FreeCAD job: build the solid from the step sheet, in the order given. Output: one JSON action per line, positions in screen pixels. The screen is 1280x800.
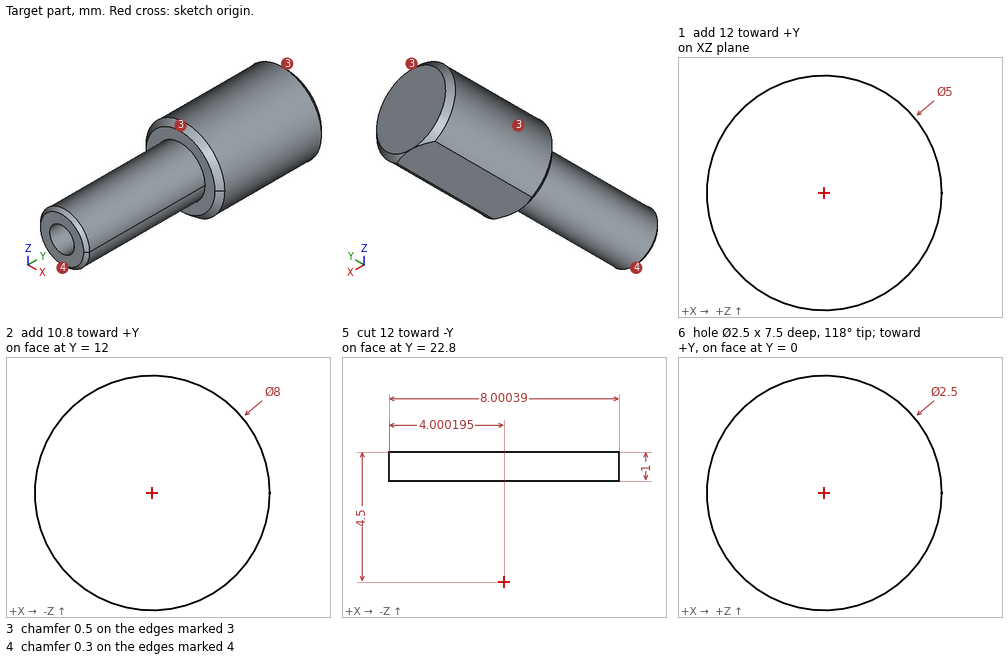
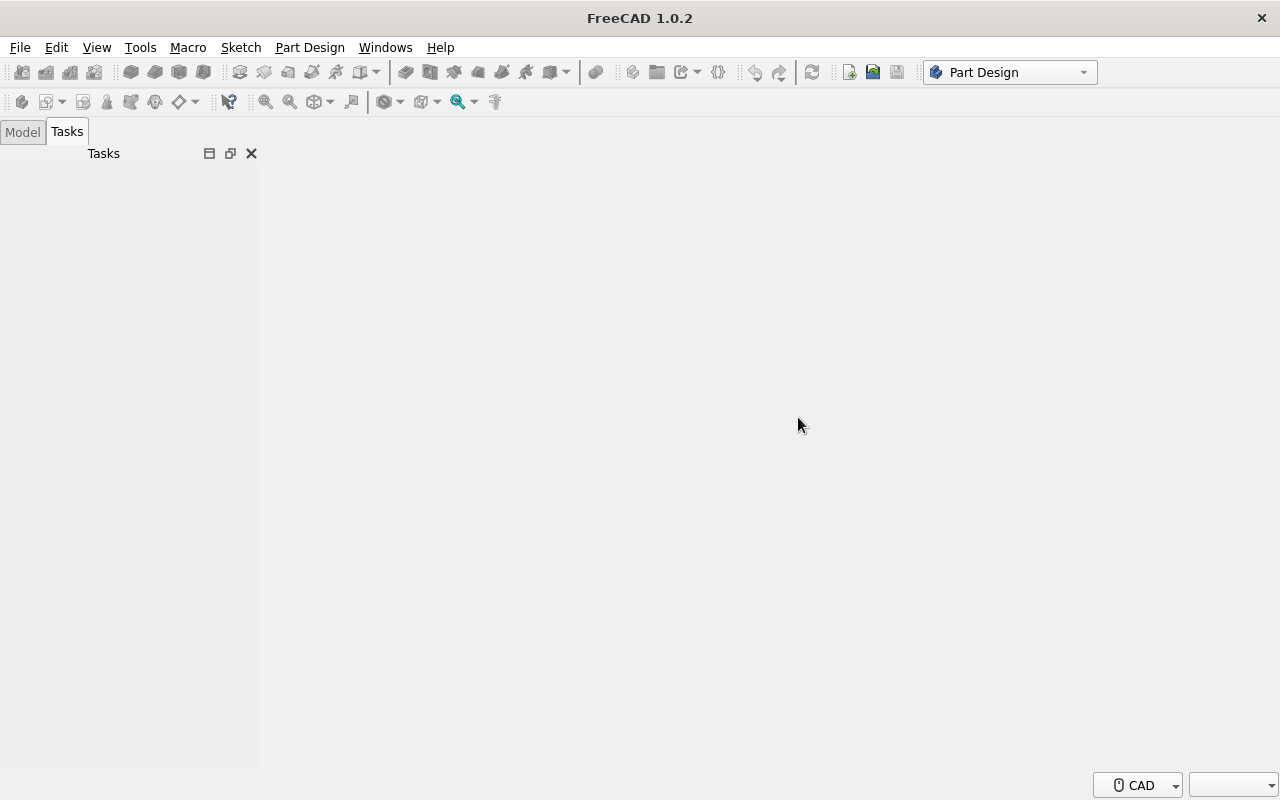
{"action": "left_click", "coordinate": [850, 72]}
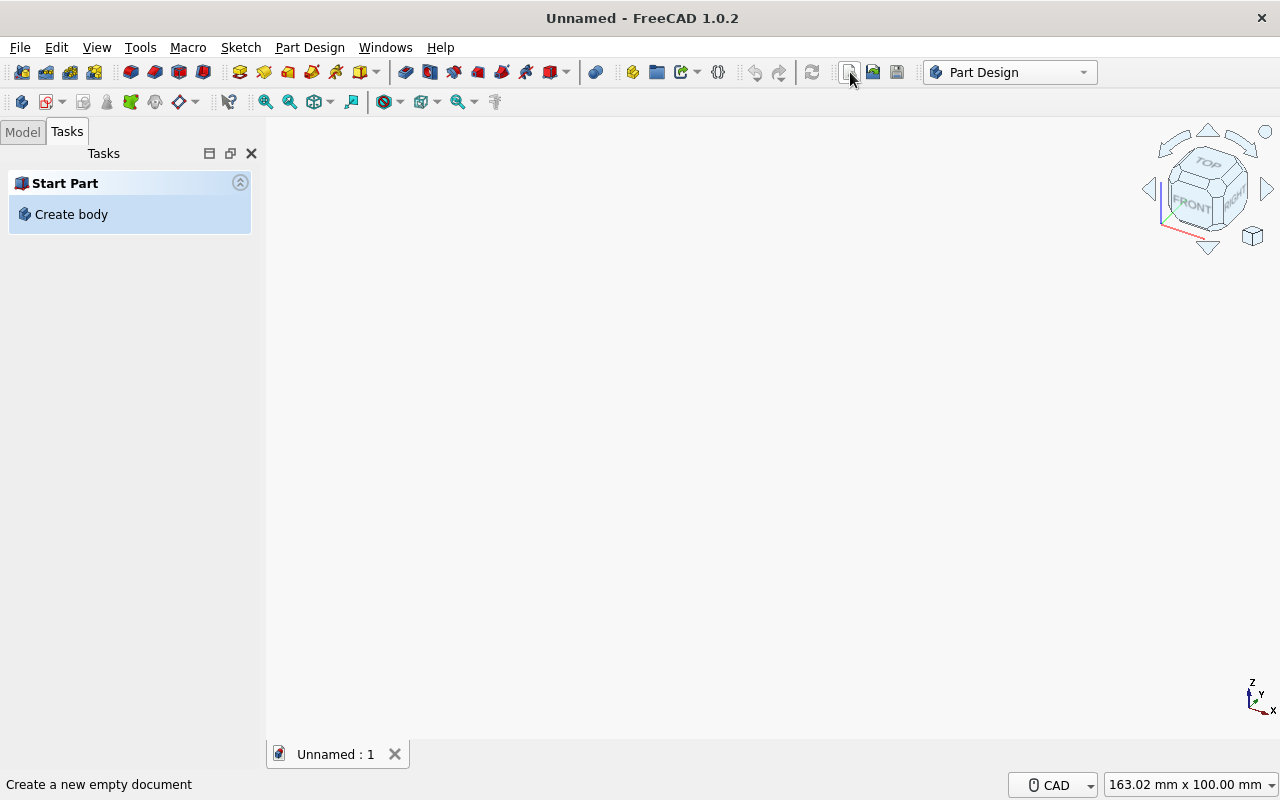
{"action": "left_click", "coordinate": [46, 102]}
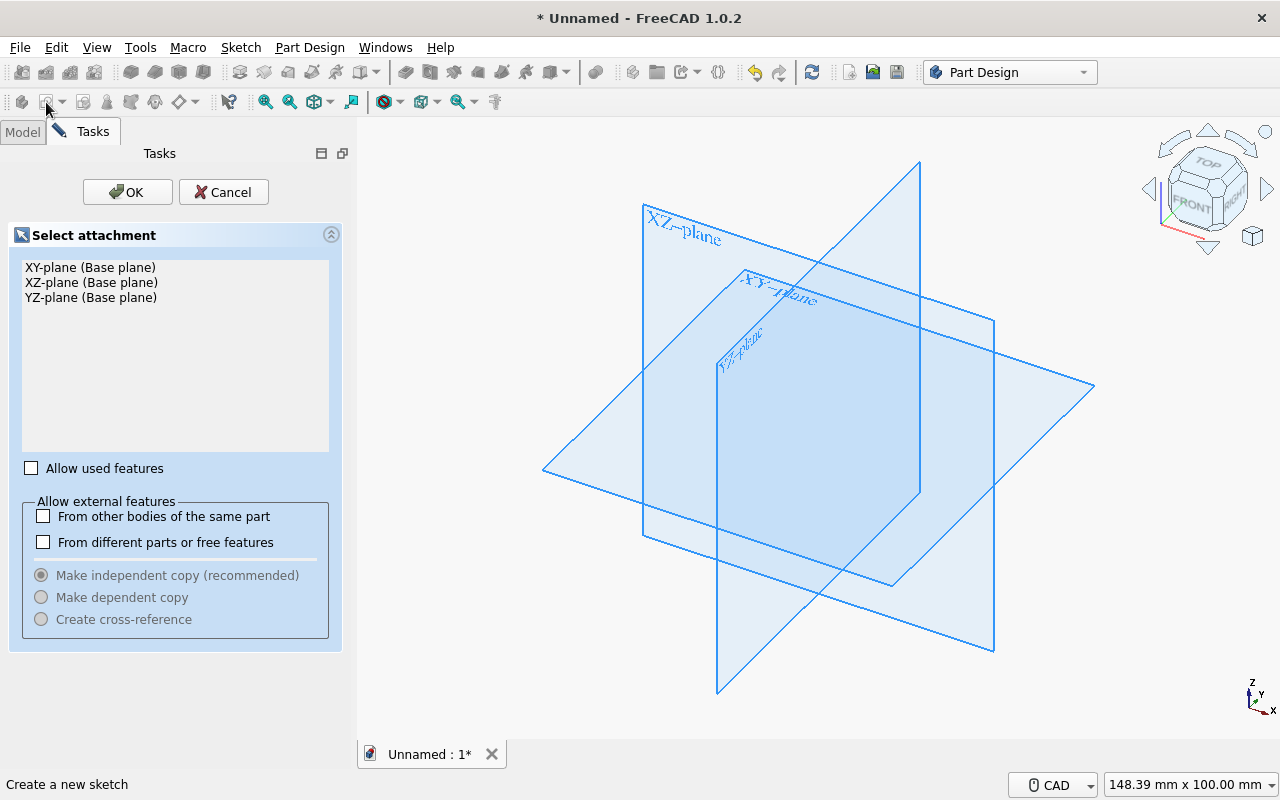
{"action": "left_click", "coordinate": [82, 282]}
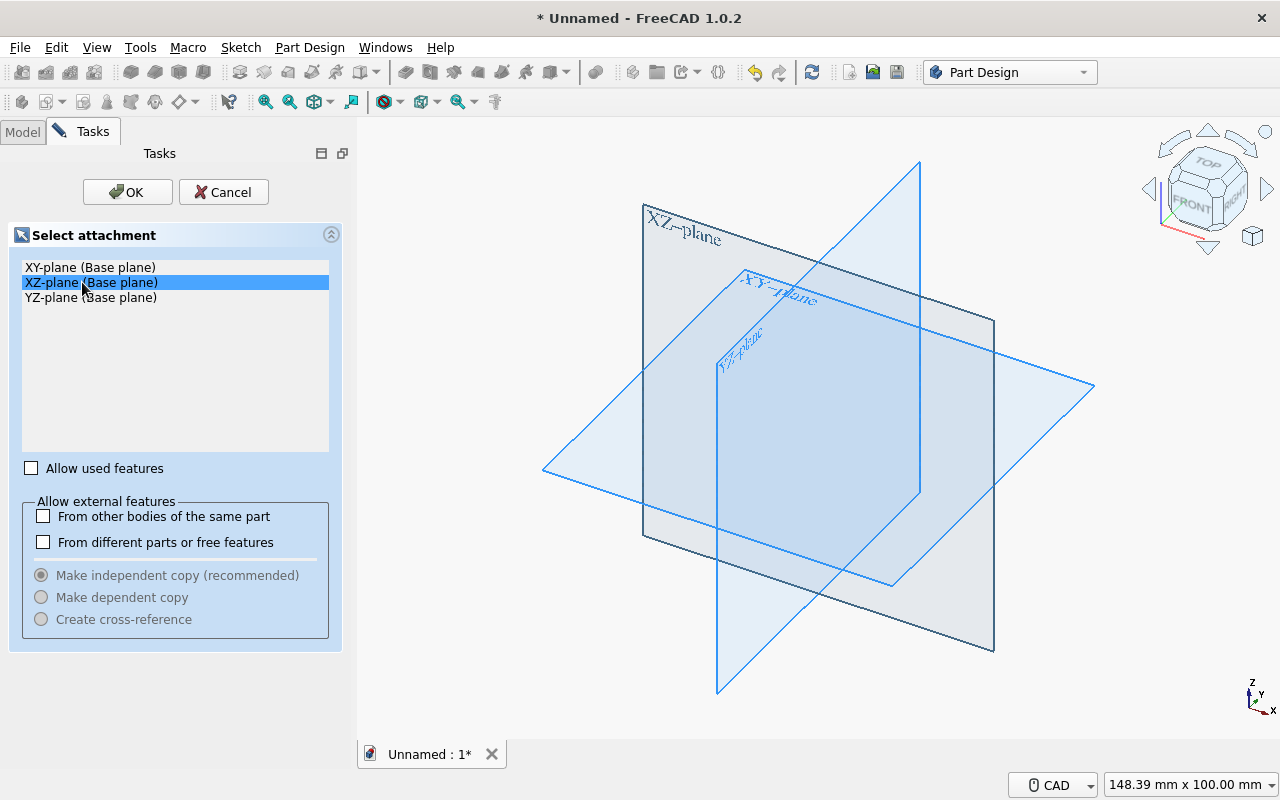
{"action": "left_click", "coordinate": [128, 192]}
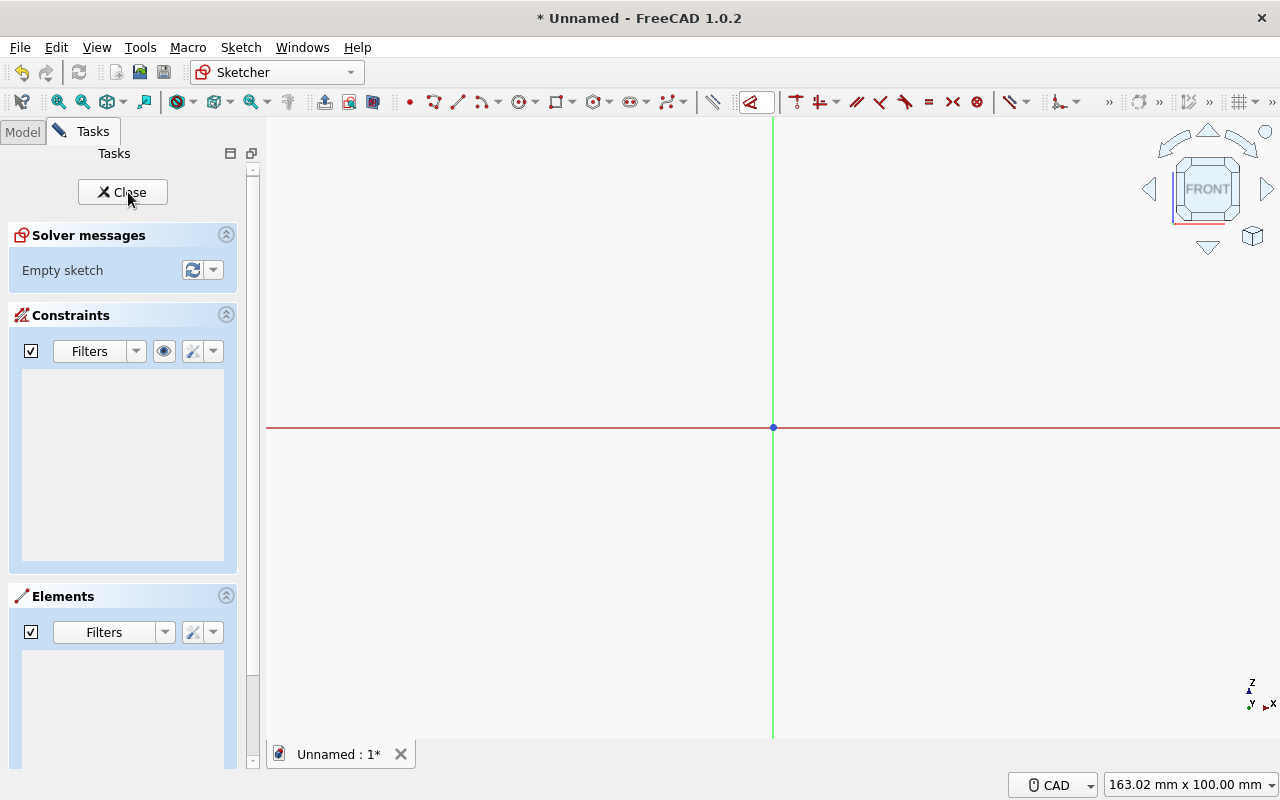
{"action": "scroll", "coordinate": [778, 428], "scroll_direction": "up", "scroll_amount": 13}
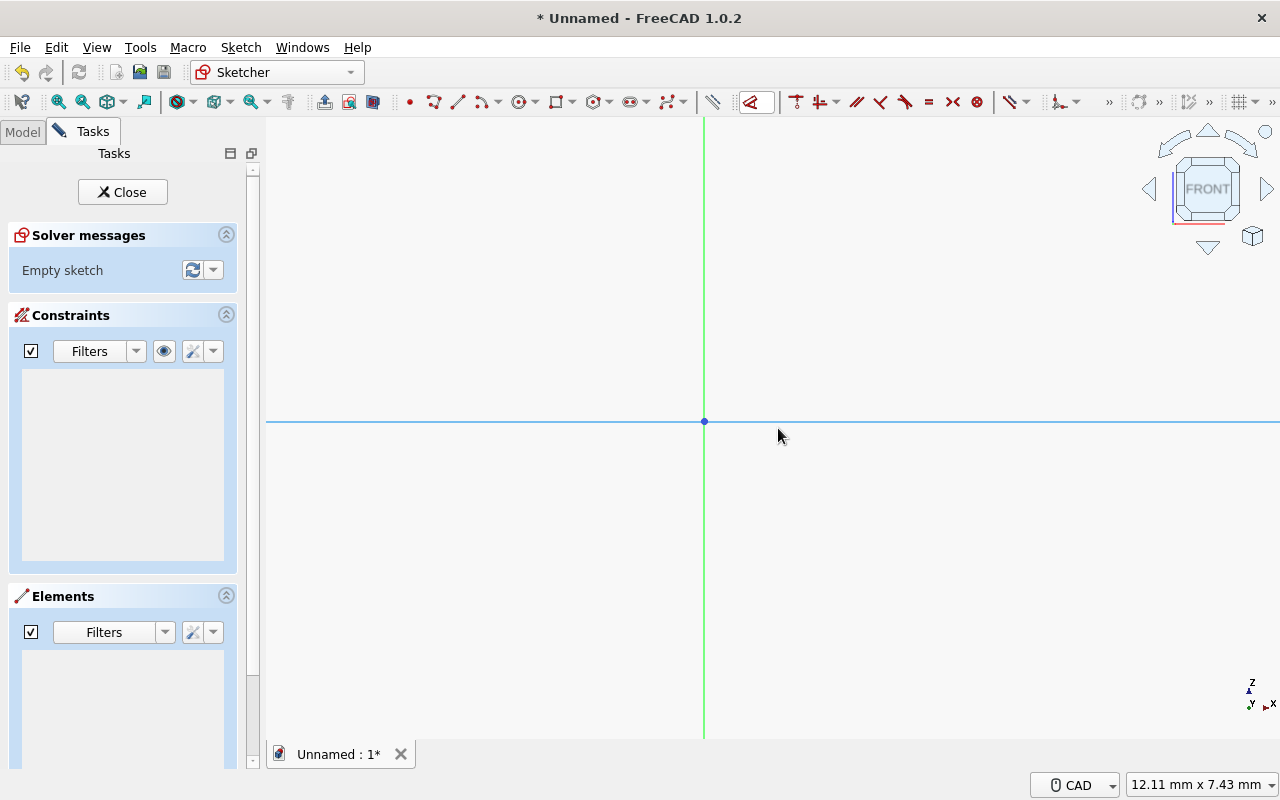
{"action": "key", "text": "g c"}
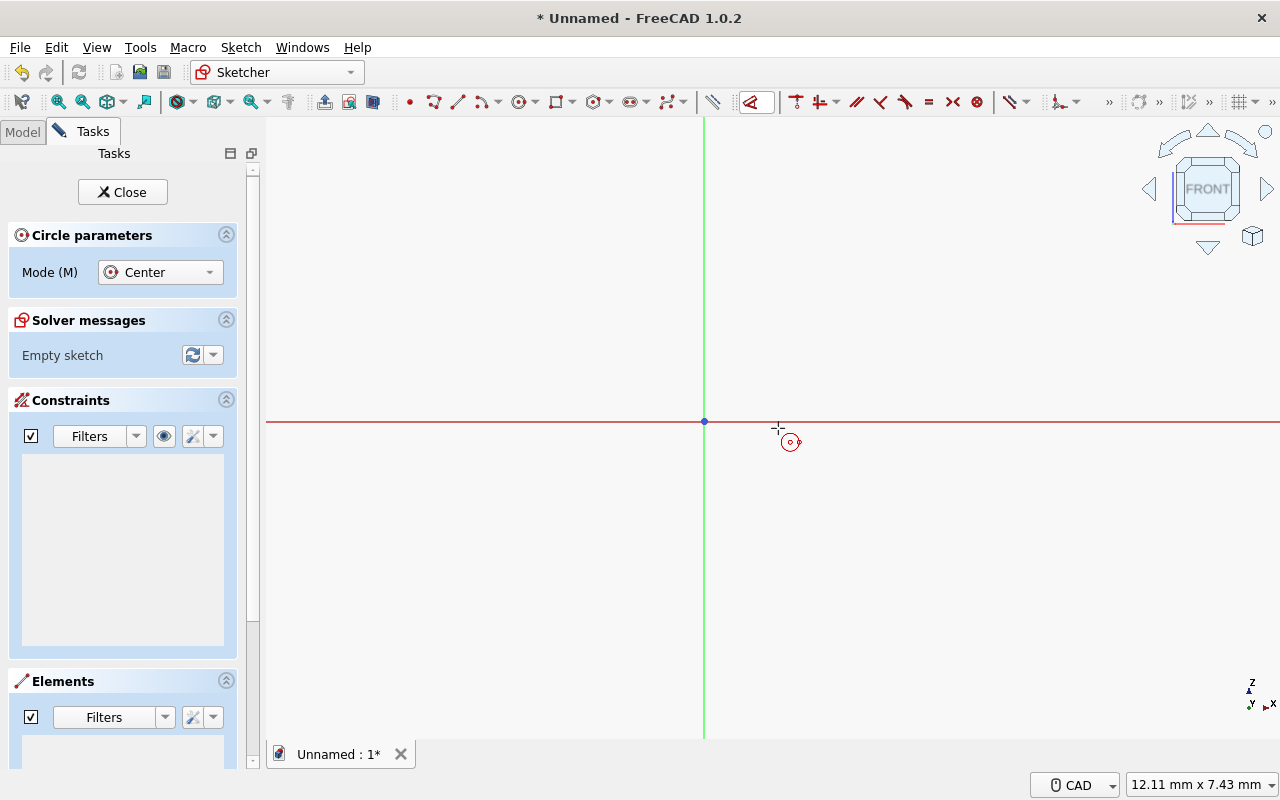
{"action": "left_click", "coordinate": [704, 422]}
{"action": "mouse_move", "coordinate": [852, 274]}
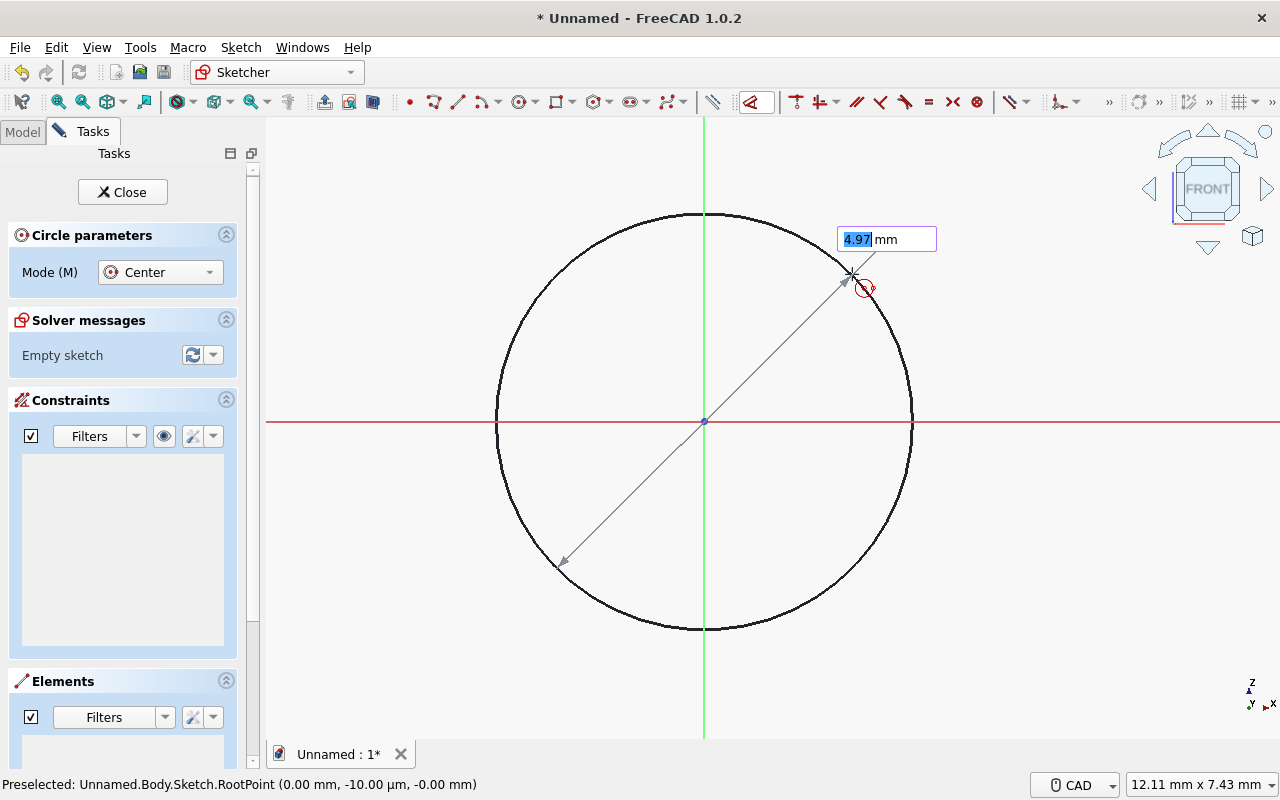
{"action": "type", "text": "5"}
{"action": "key", "text": "Return"}
{"action": "key", "text": "Escape"}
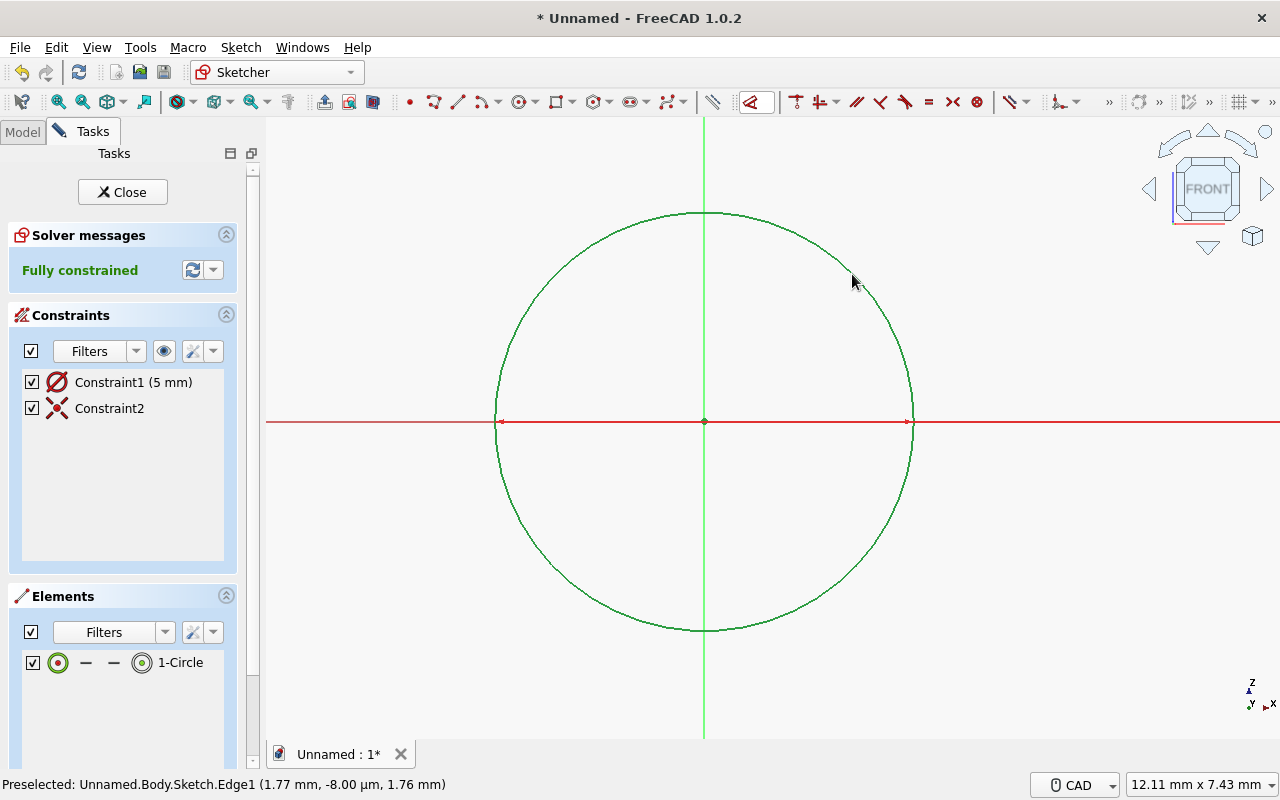
{"action": "left_click", "coordinate": [123, 192]}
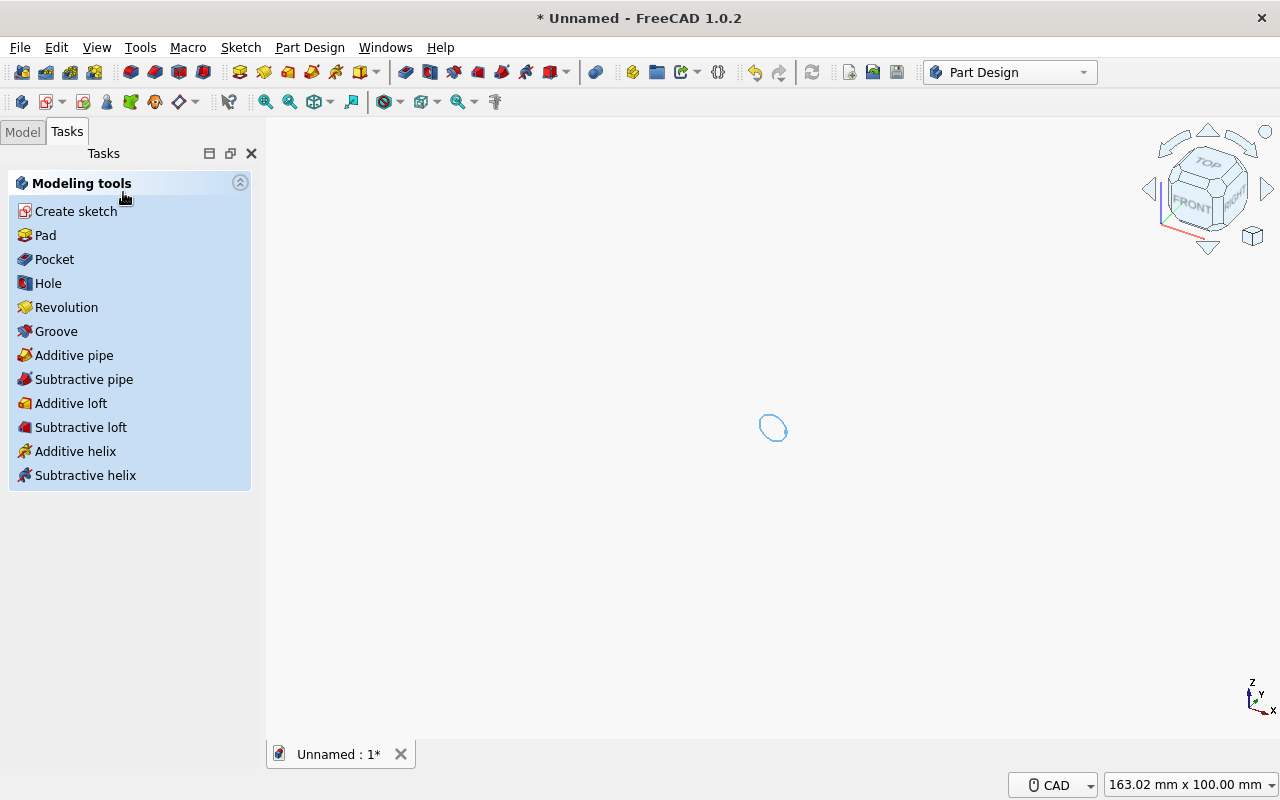
{"action": "left_click", "coordinate": [240, 72]}